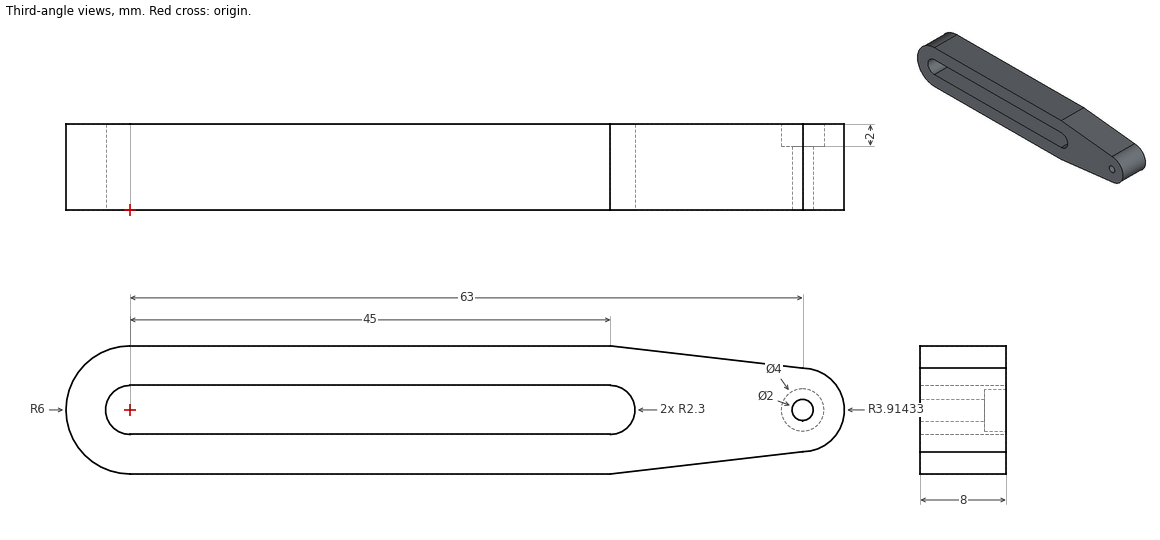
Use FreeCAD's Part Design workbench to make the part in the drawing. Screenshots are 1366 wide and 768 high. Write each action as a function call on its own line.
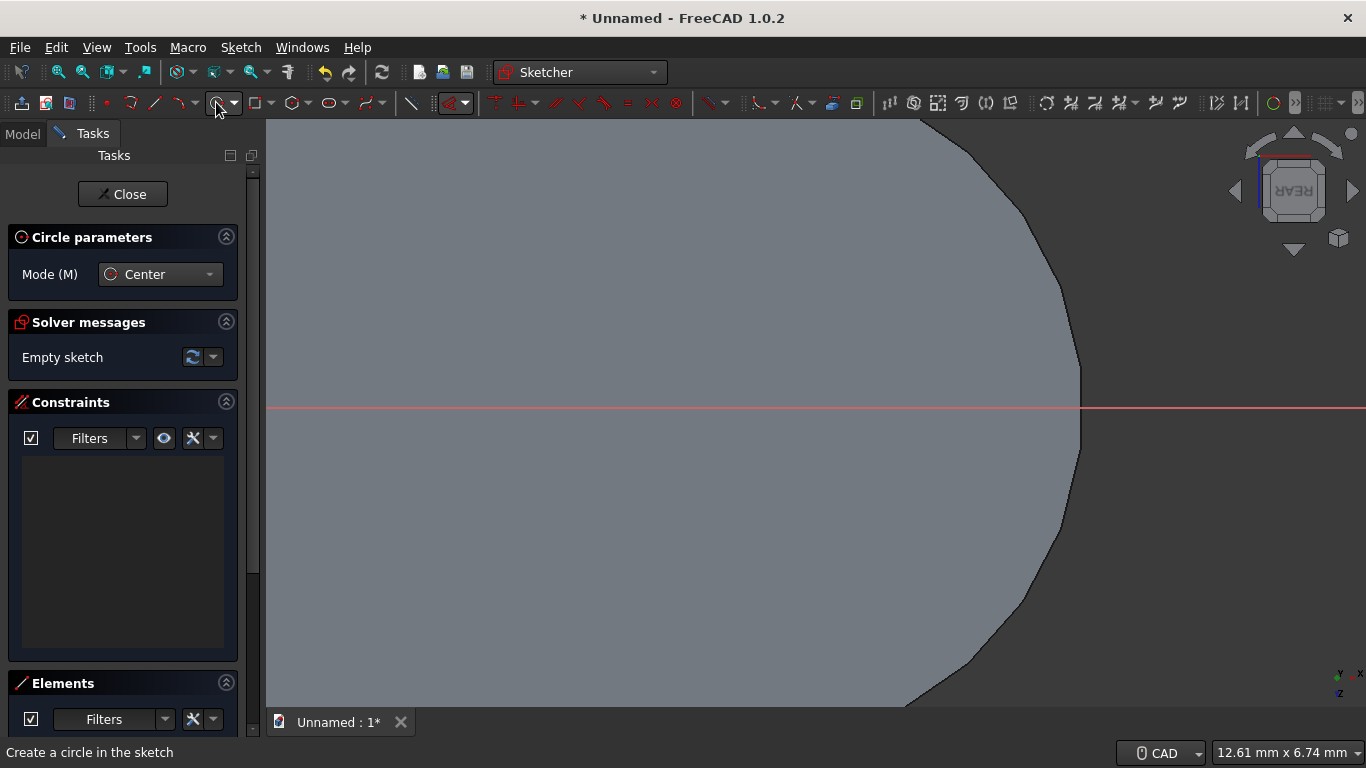
click(742, 408)
move(865, 285)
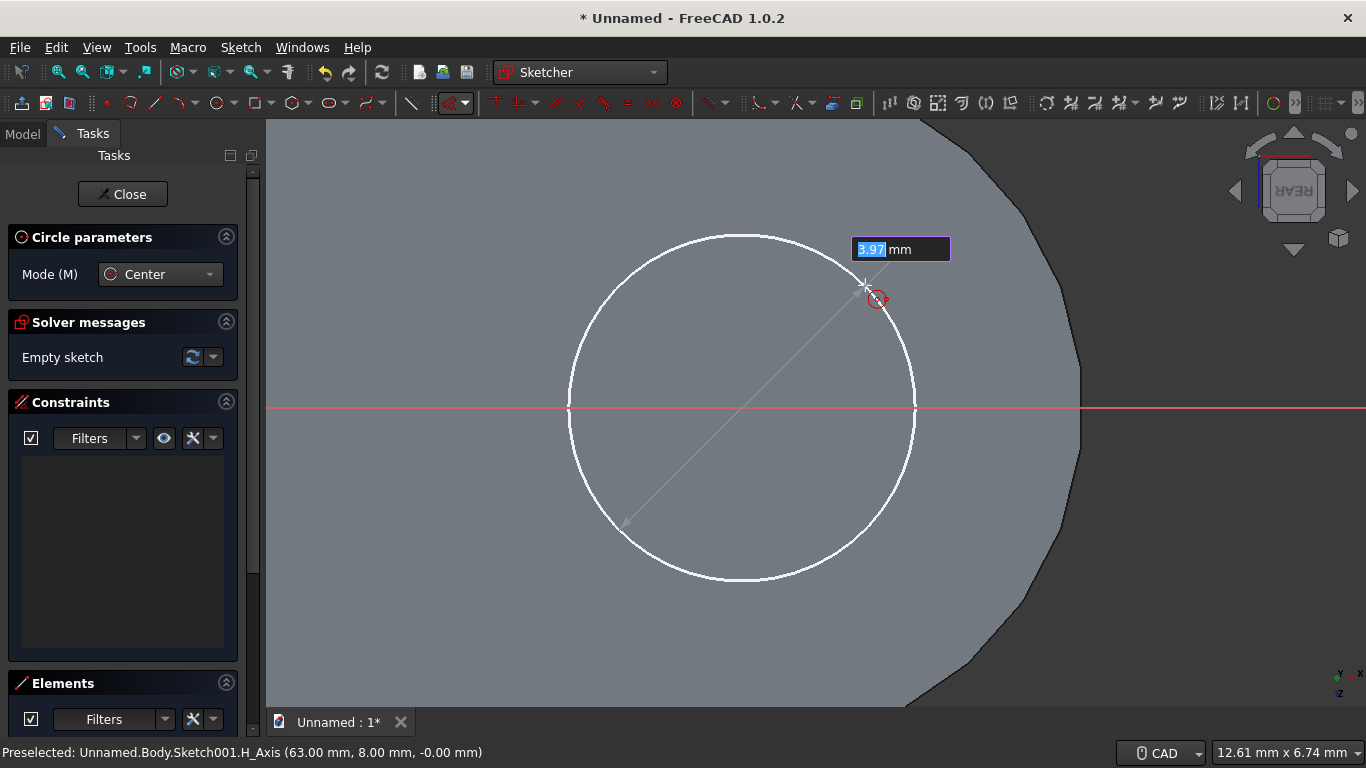
text(4)
key(Return)
key(Escape)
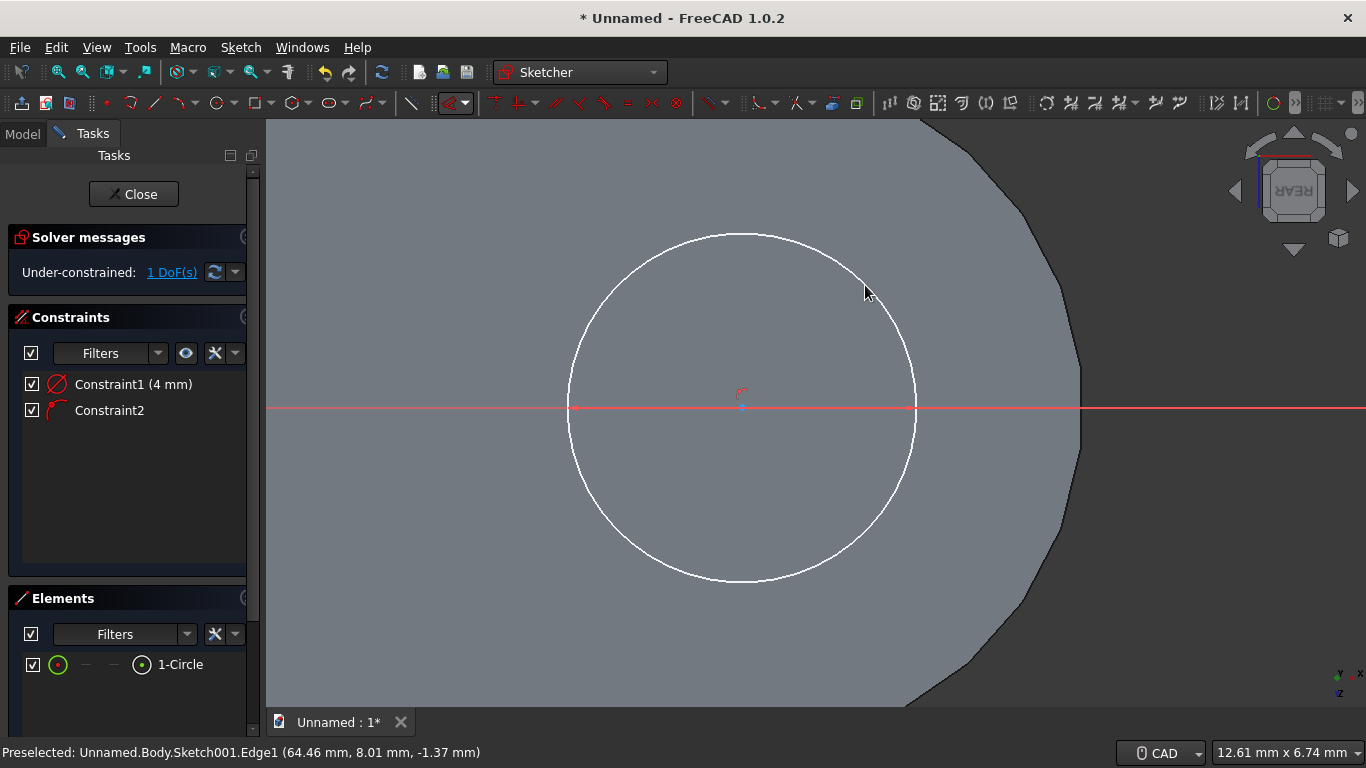
click(742, 408)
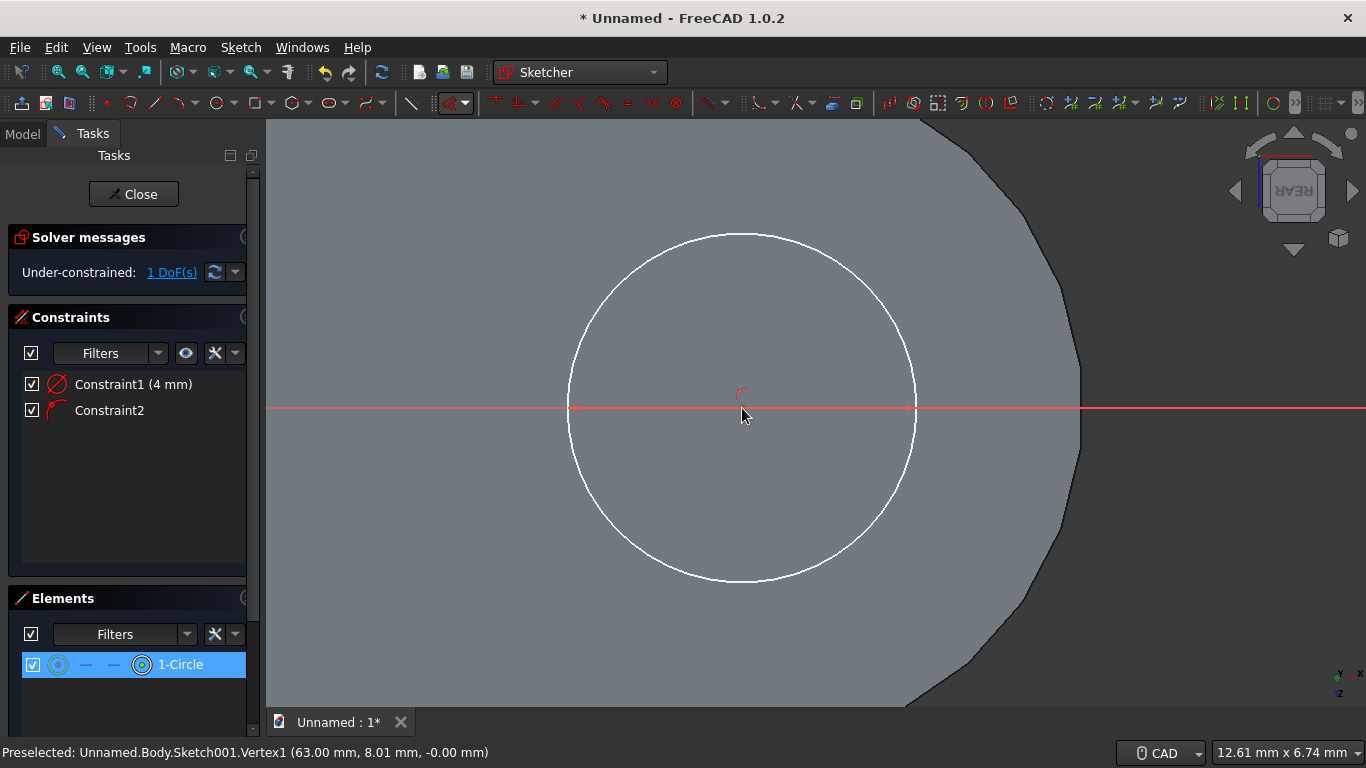
key(l)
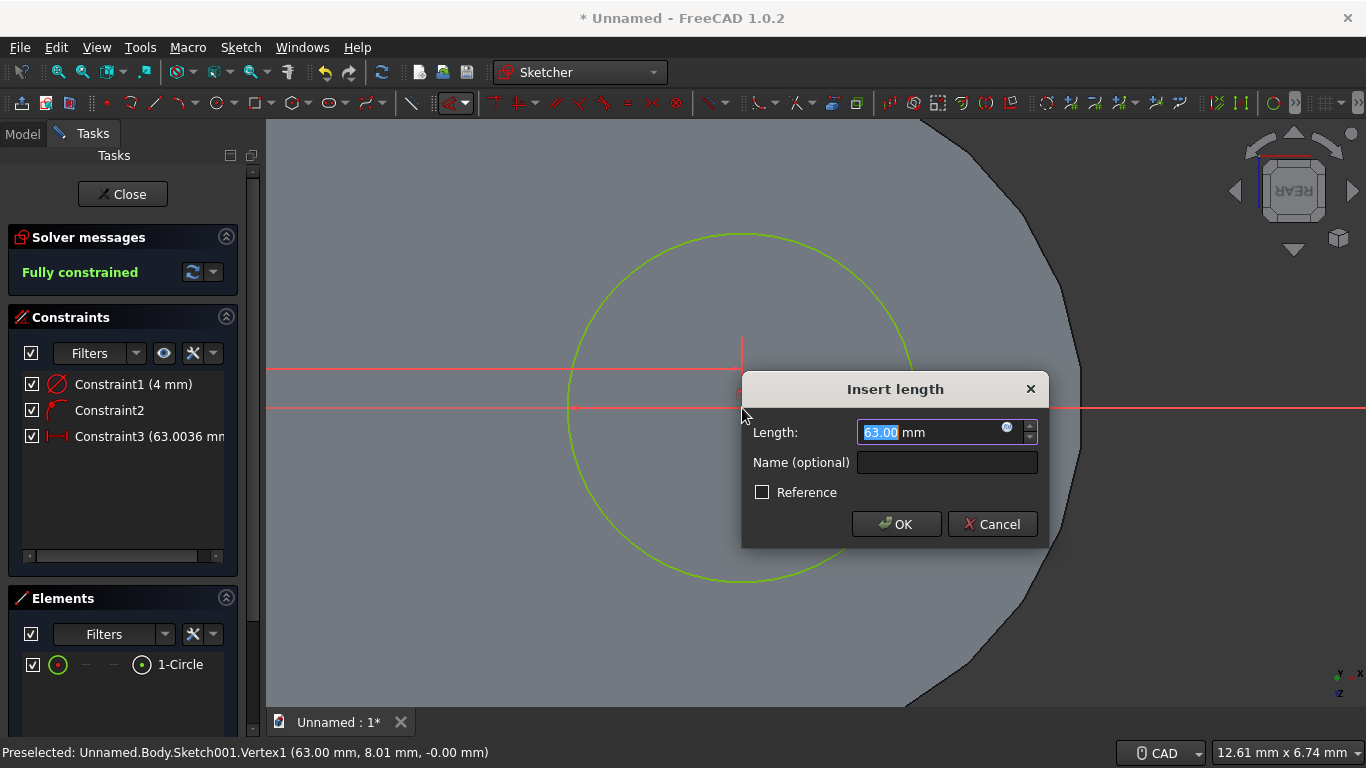
text(63)
key(Return)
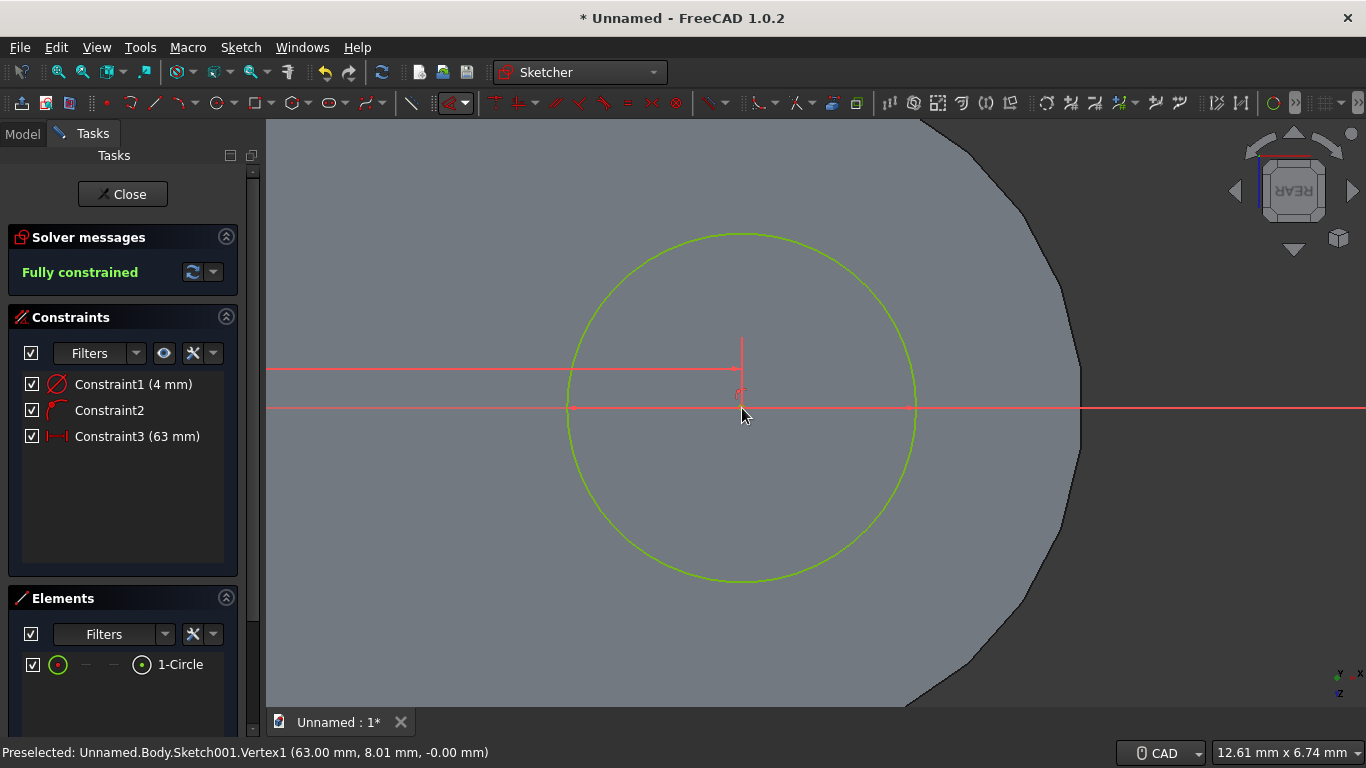
click(123, 194)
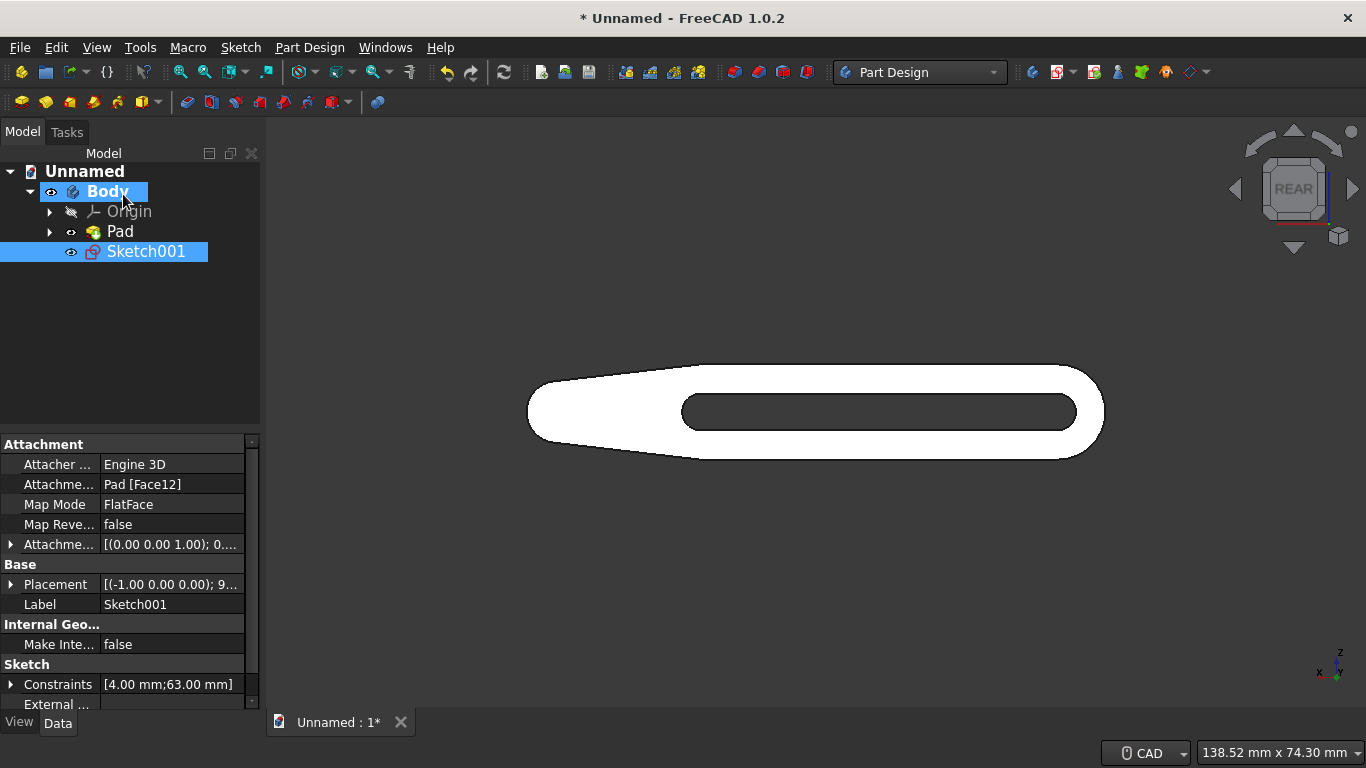
click(188, 102)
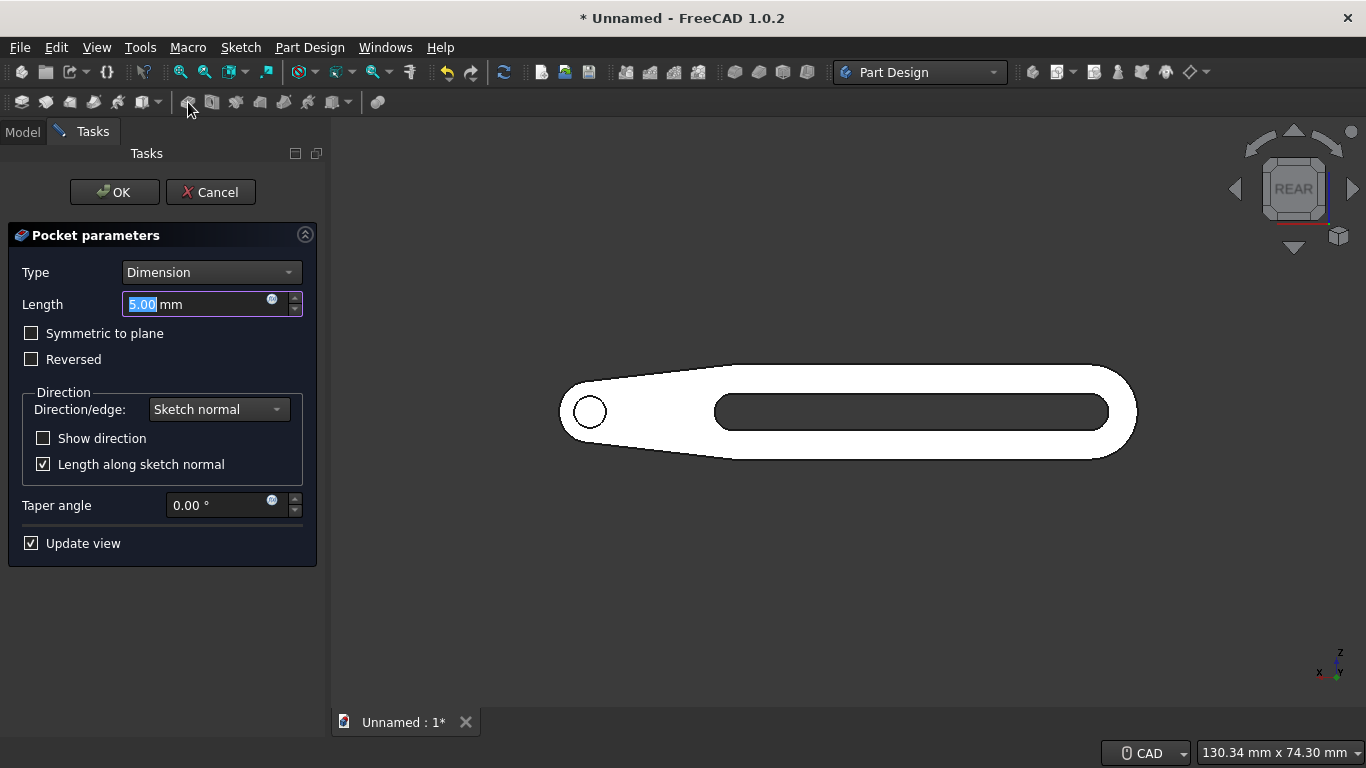
text(2)
key(Tab)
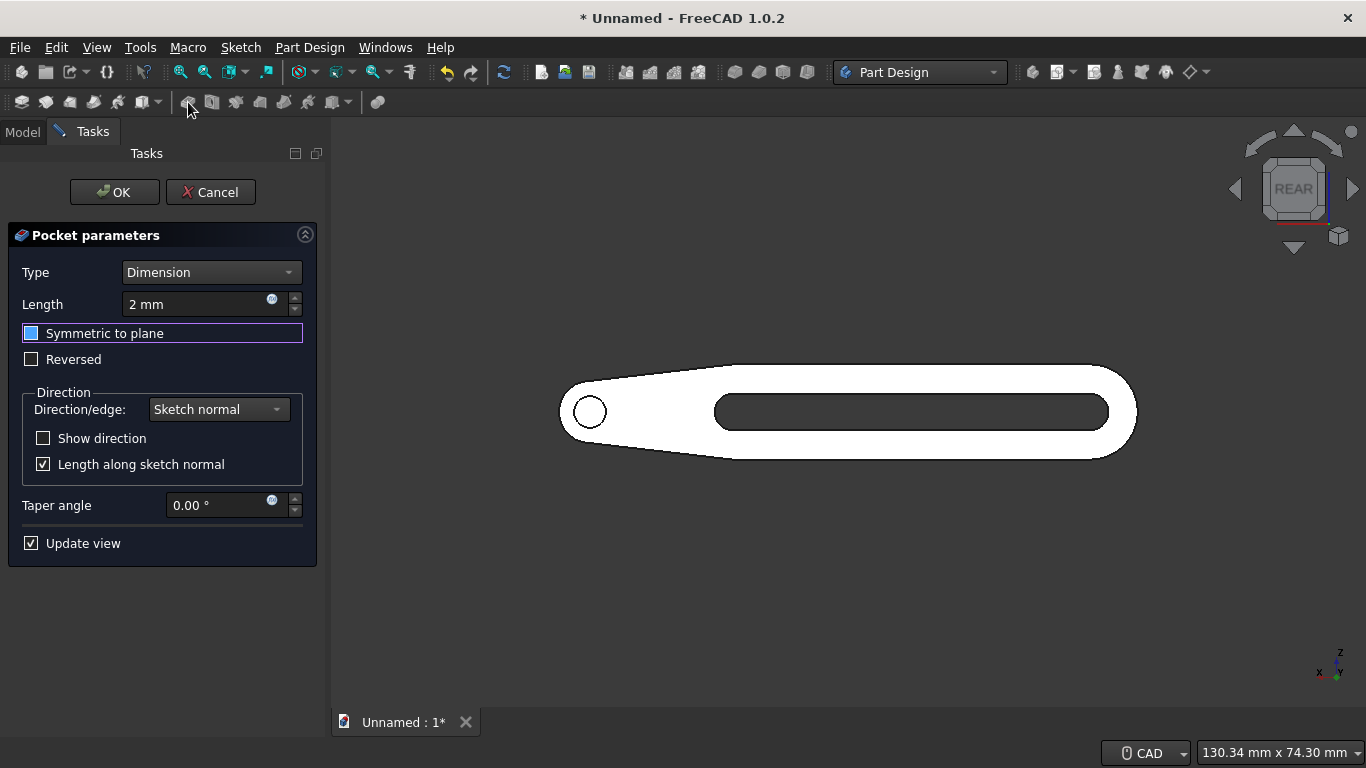
click(115, 192)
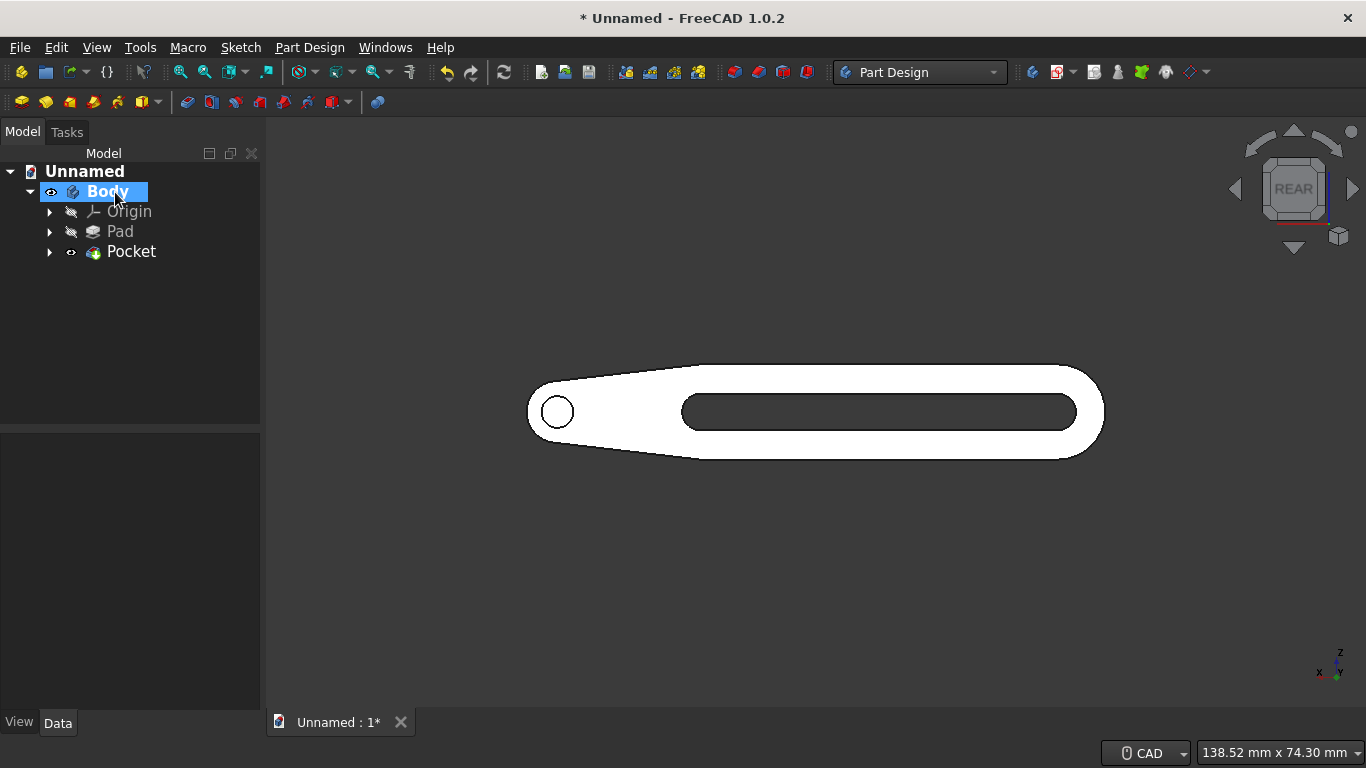
key(0)